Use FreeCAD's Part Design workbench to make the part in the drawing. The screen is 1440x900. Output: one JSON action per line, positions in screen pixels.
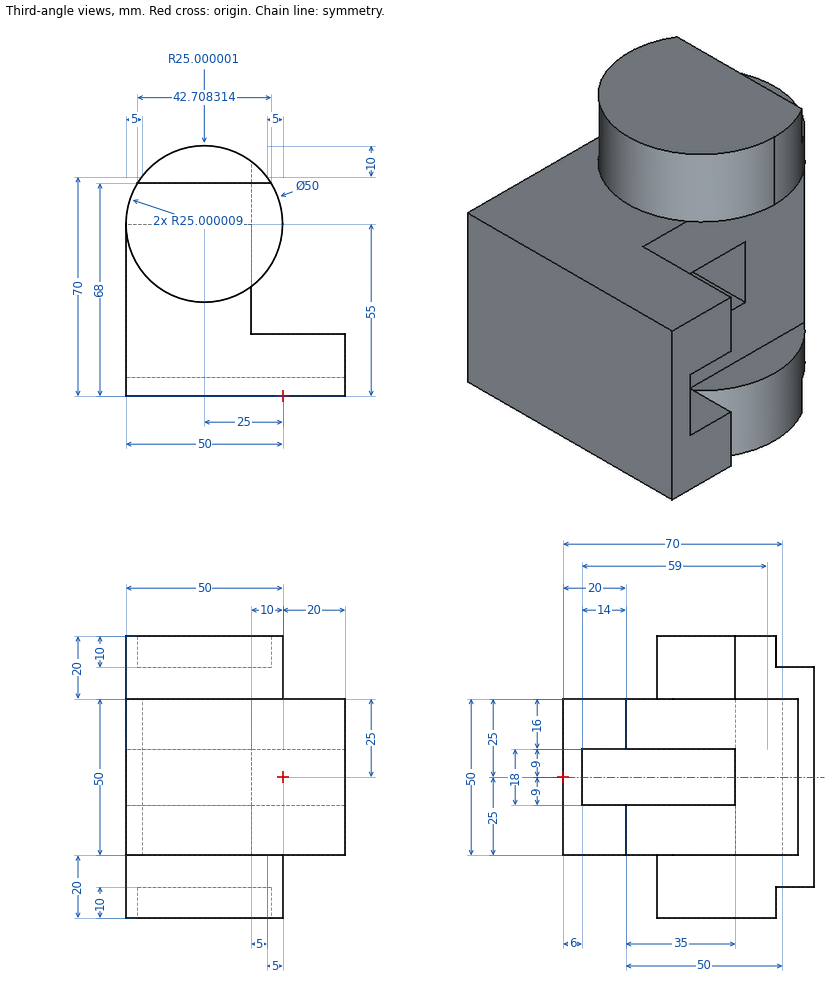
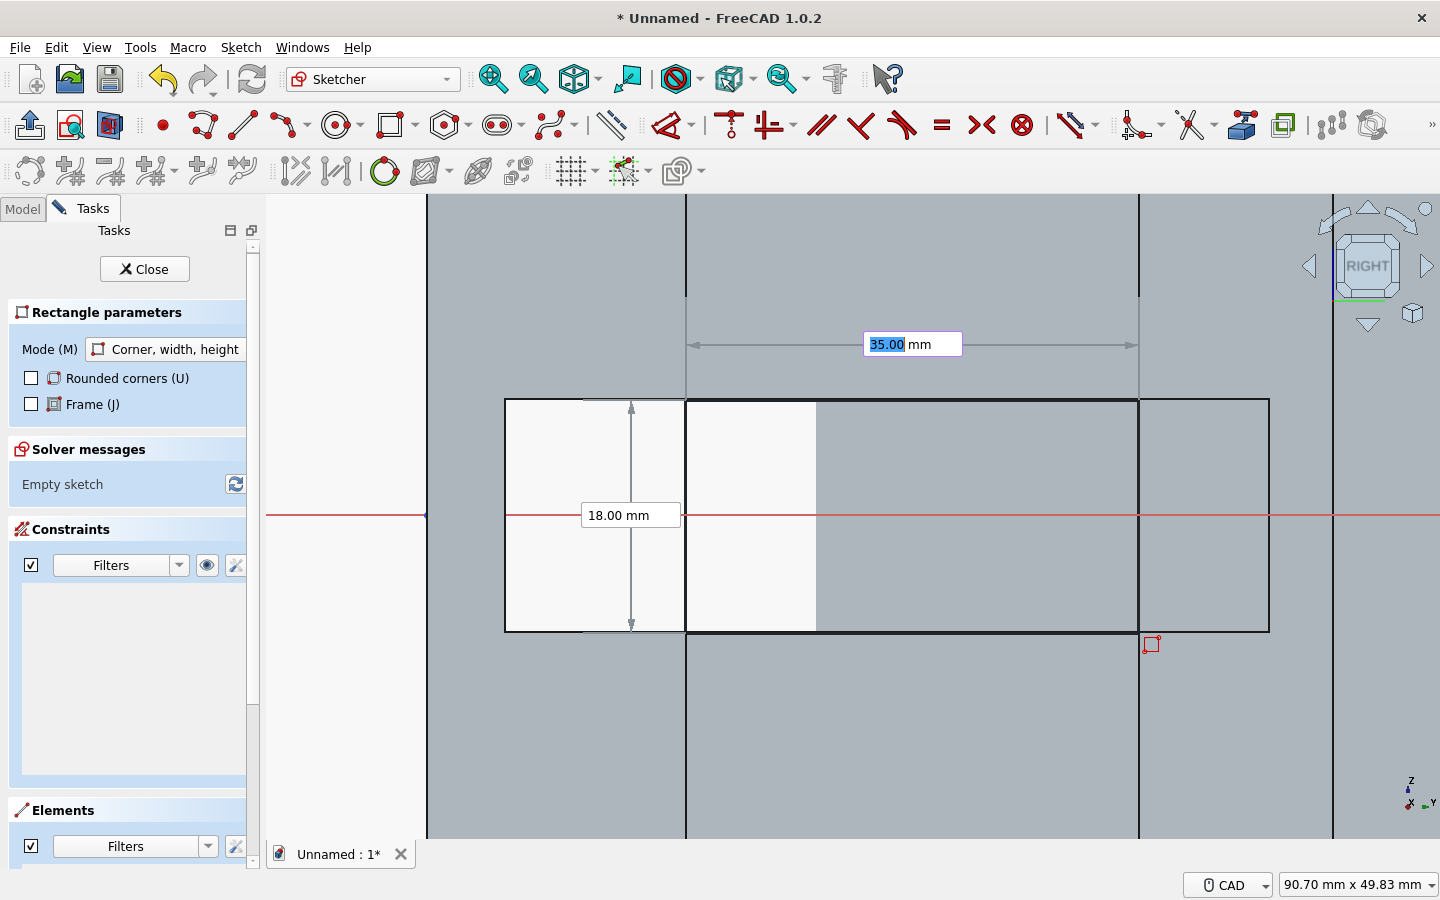
{"action": "type", "text": "35"}
{"action": "key", "text": "Tab"}
{"action": "type", "text": "18"}
{"action": "key", "text": "Return"}
{"action": "key", "text": "Escape"}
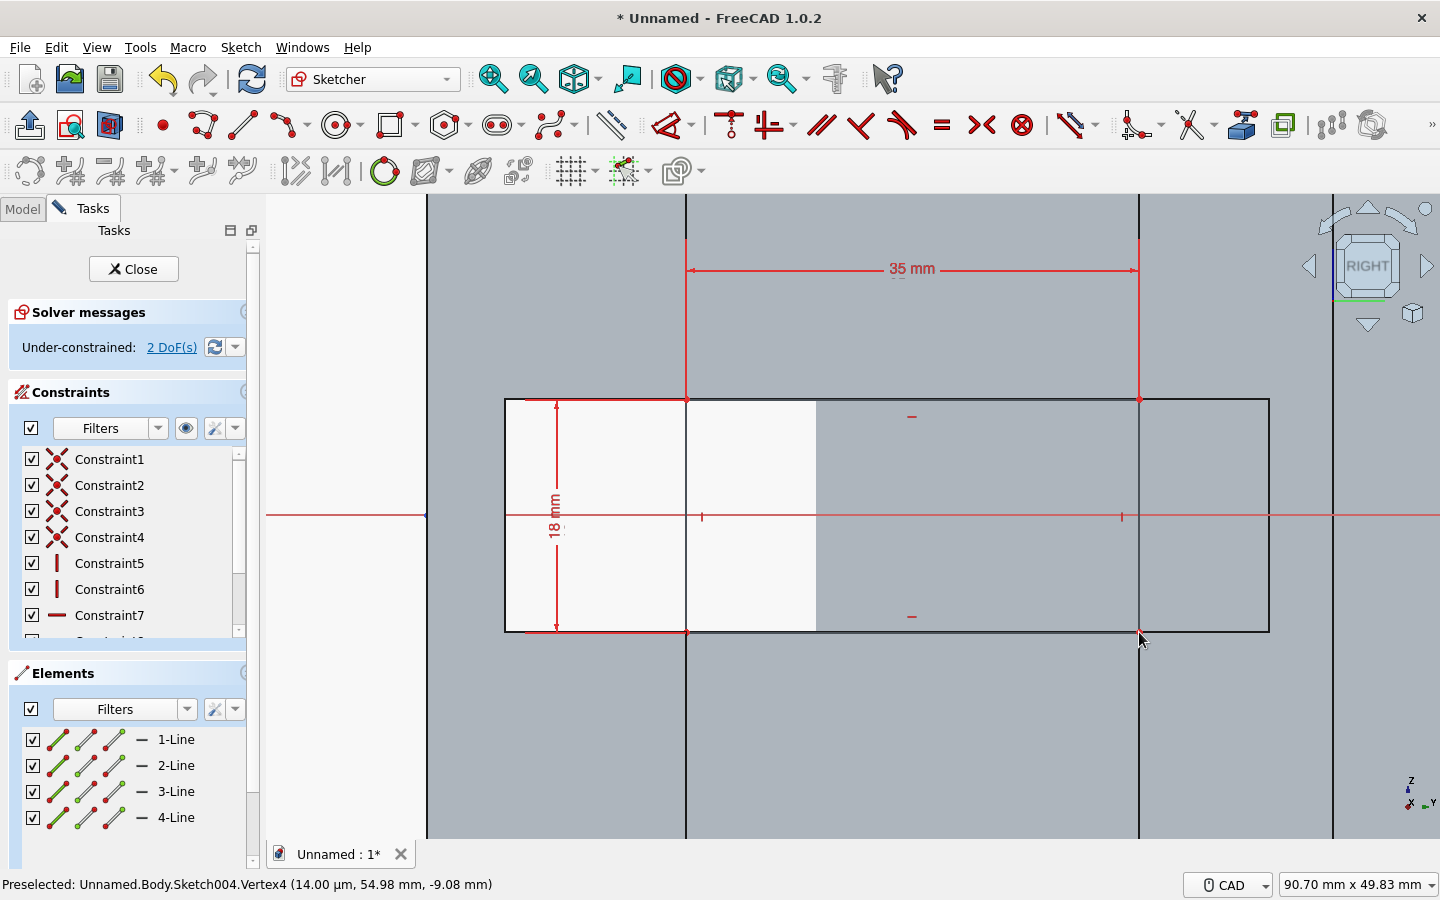
{"action": "key", "text": "d"}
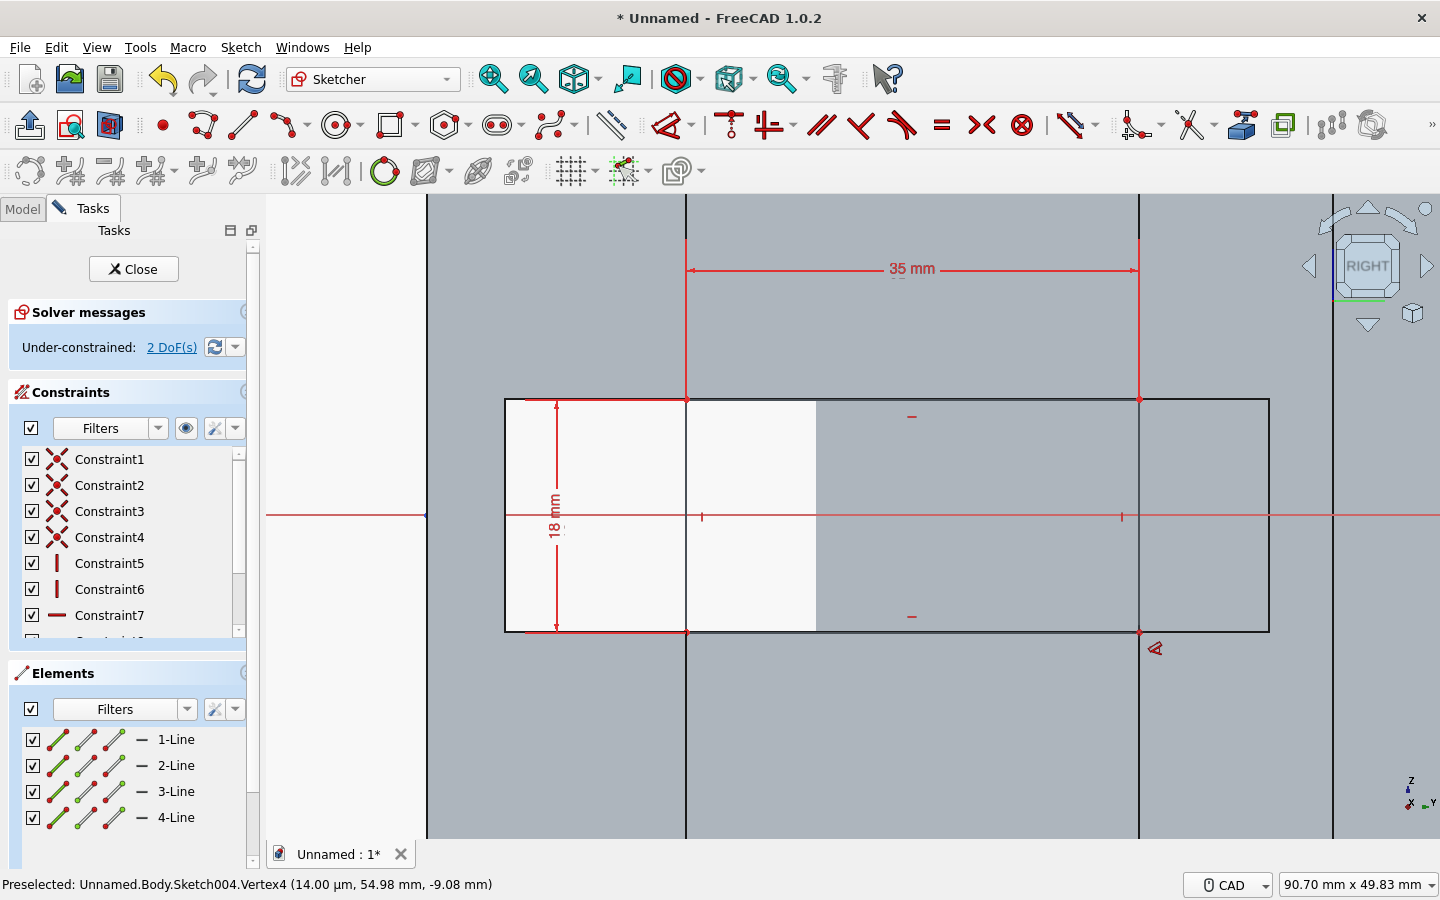
{"action": "left_click", "coordinate": [686, 400]}
{"action": "left_click", "coordinate": [393, 458]}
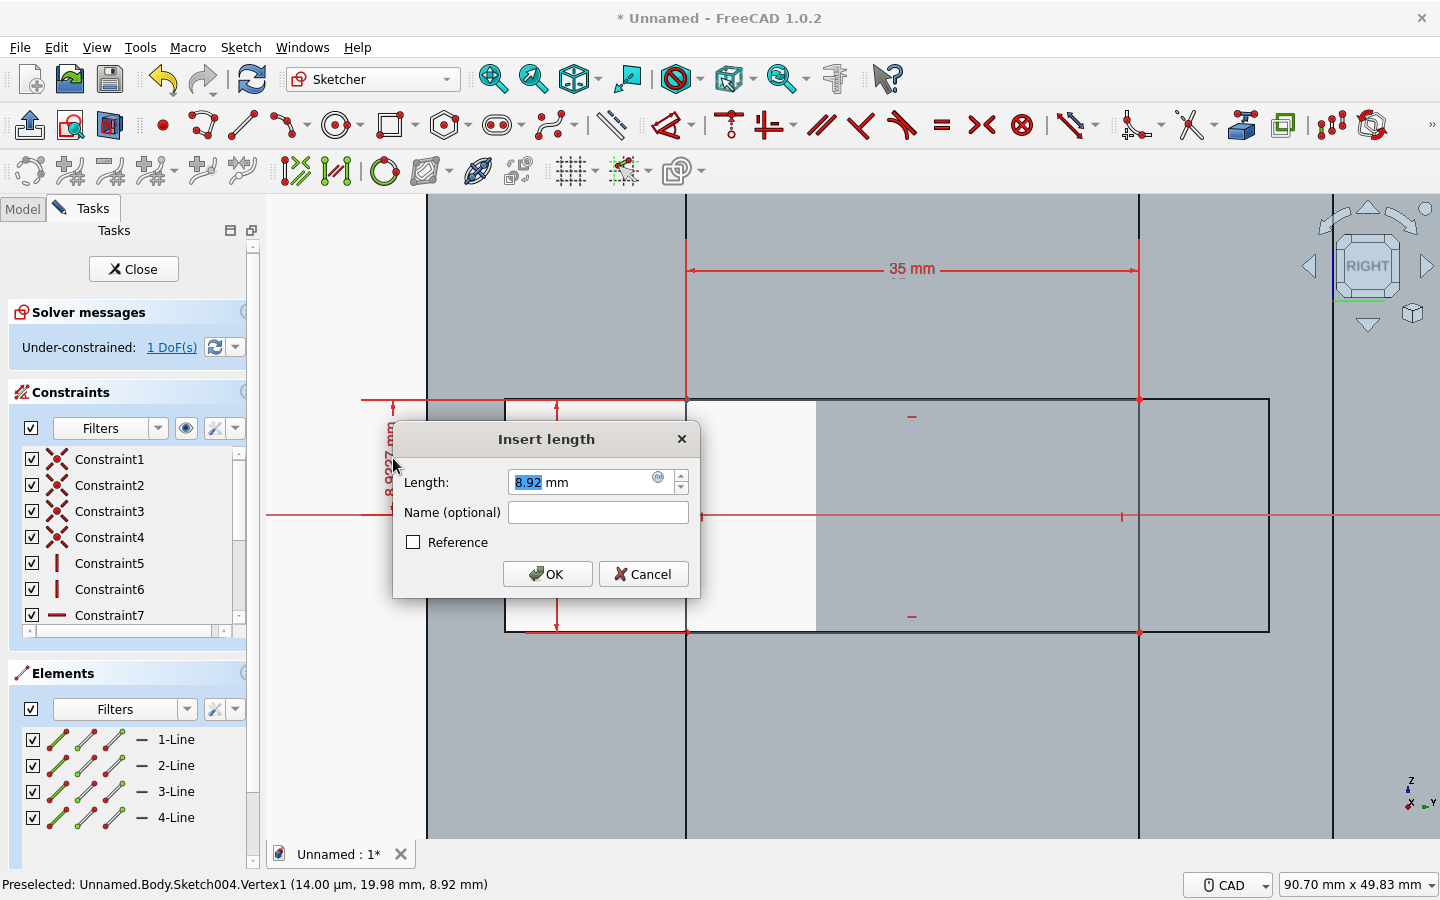
{"action": "type", "text": "9"}
{"action": "key", "text": "Return"}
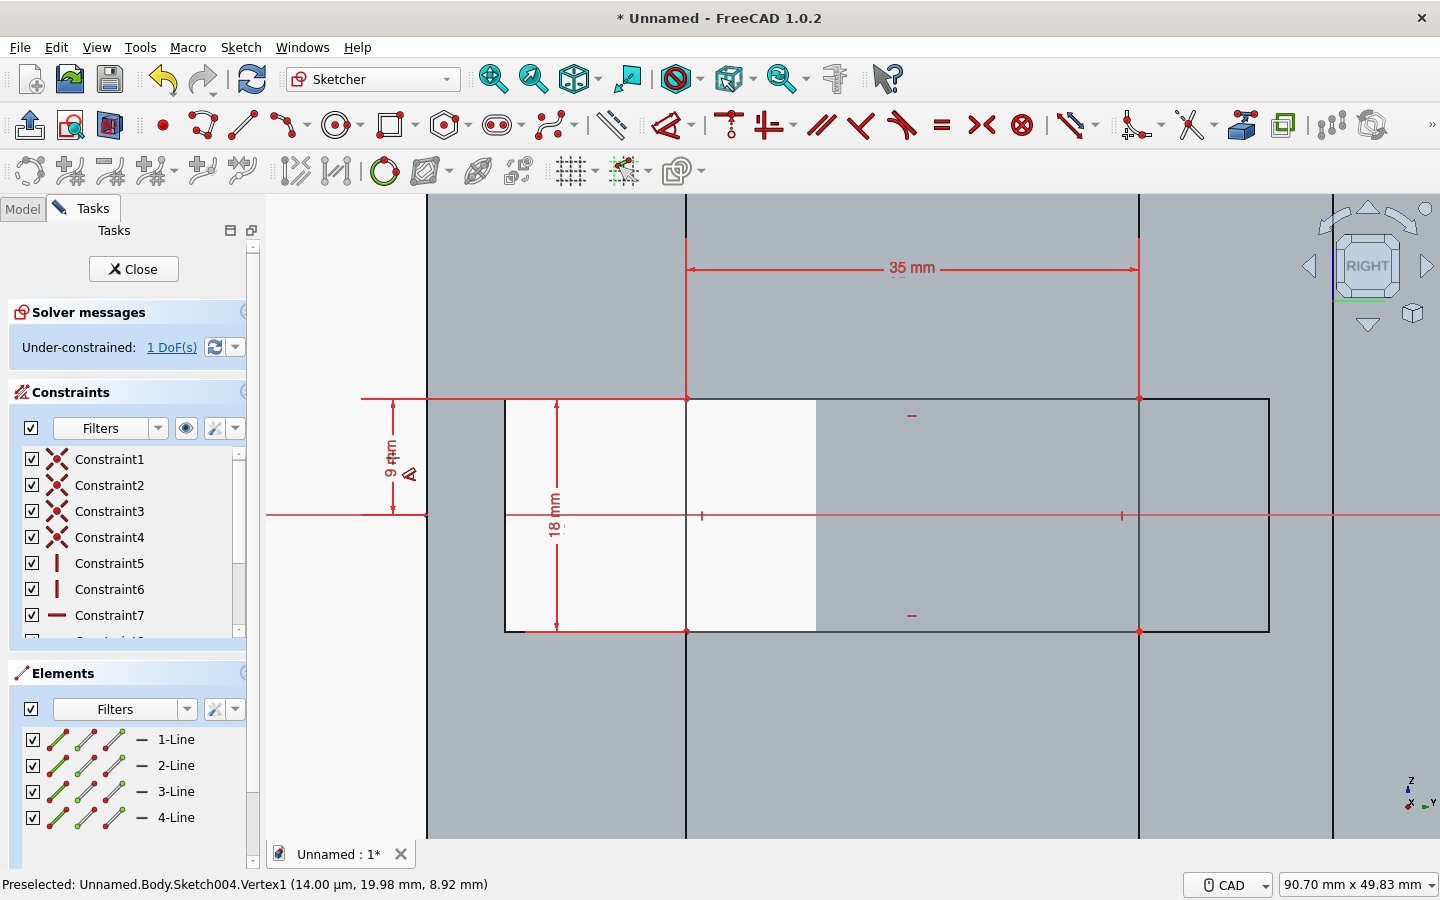
{"action": "left_click", "coordinate": [686, 399]}
{"action": "left_click", "coordinate": [557, 365]}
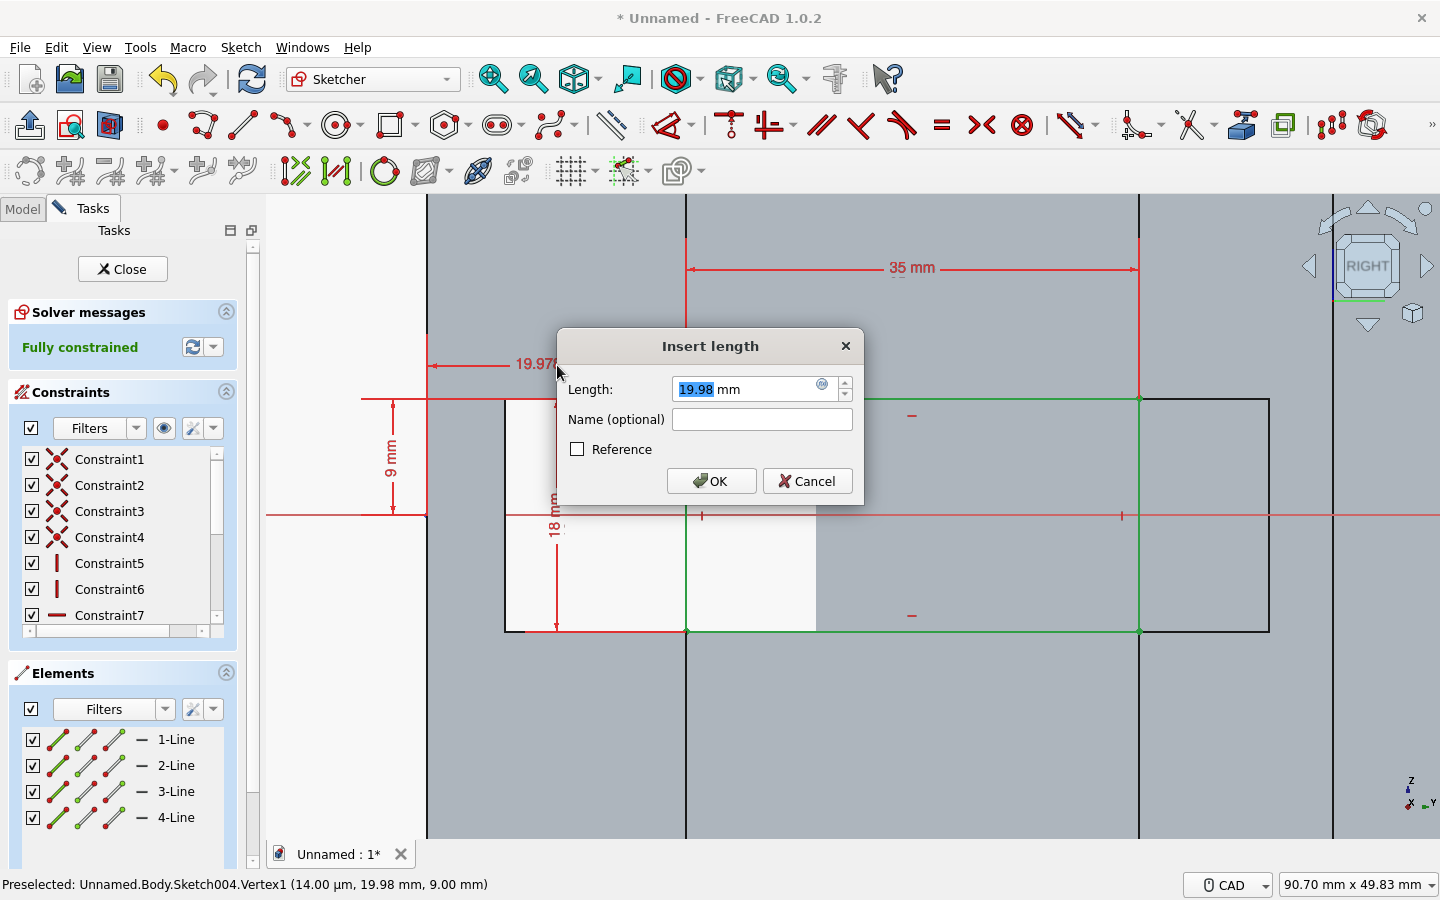
{"action": "type", "text": "20"}
{"action": "key", "text": "Return"}
{"action": "key", "text": "Escape"}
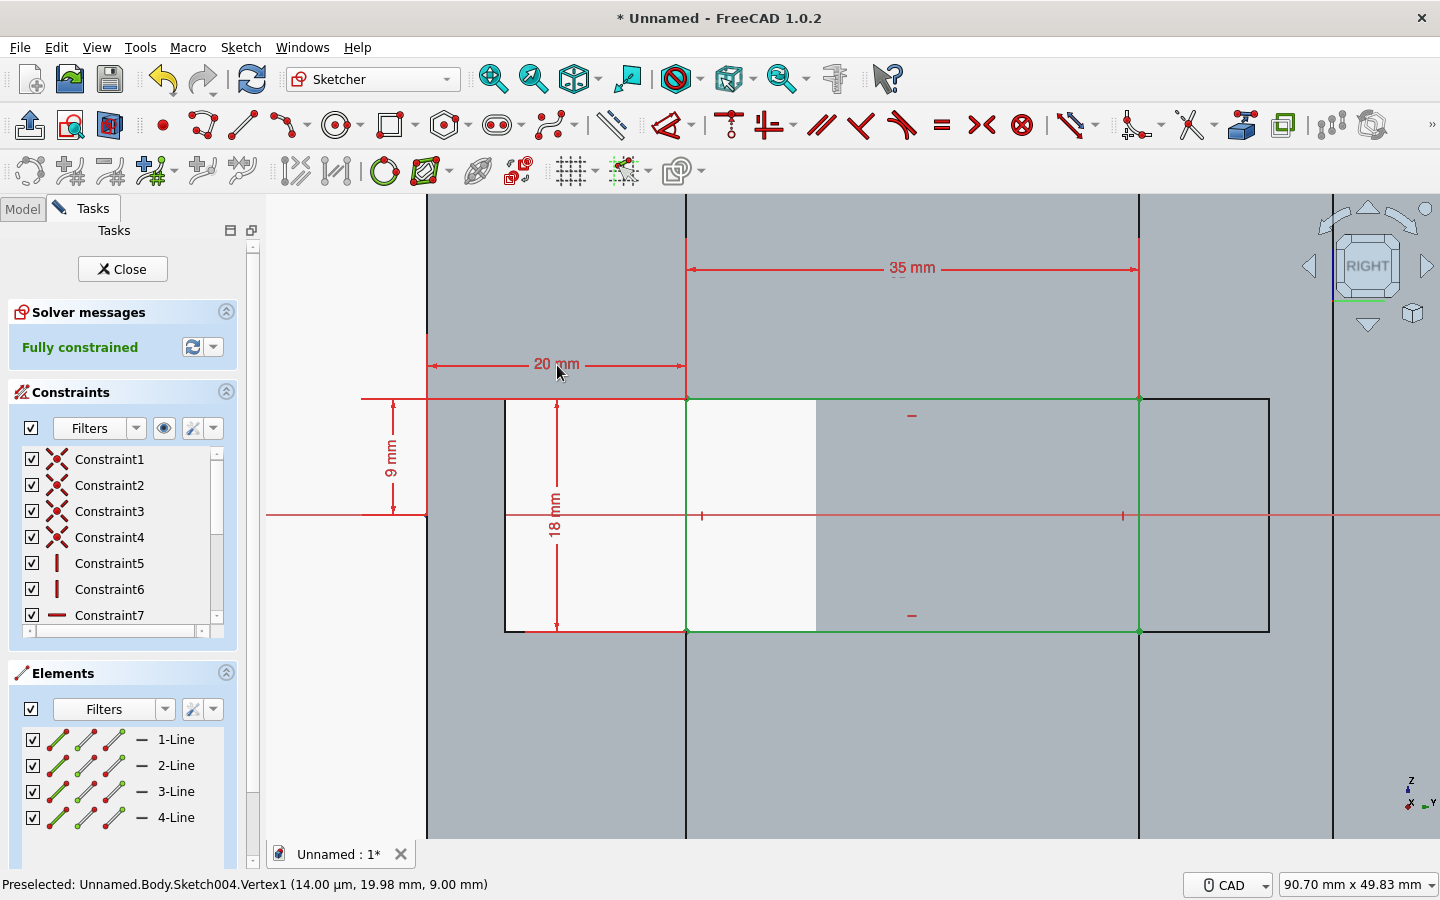
{"action": "left_click", "coordinate": [123, 269]}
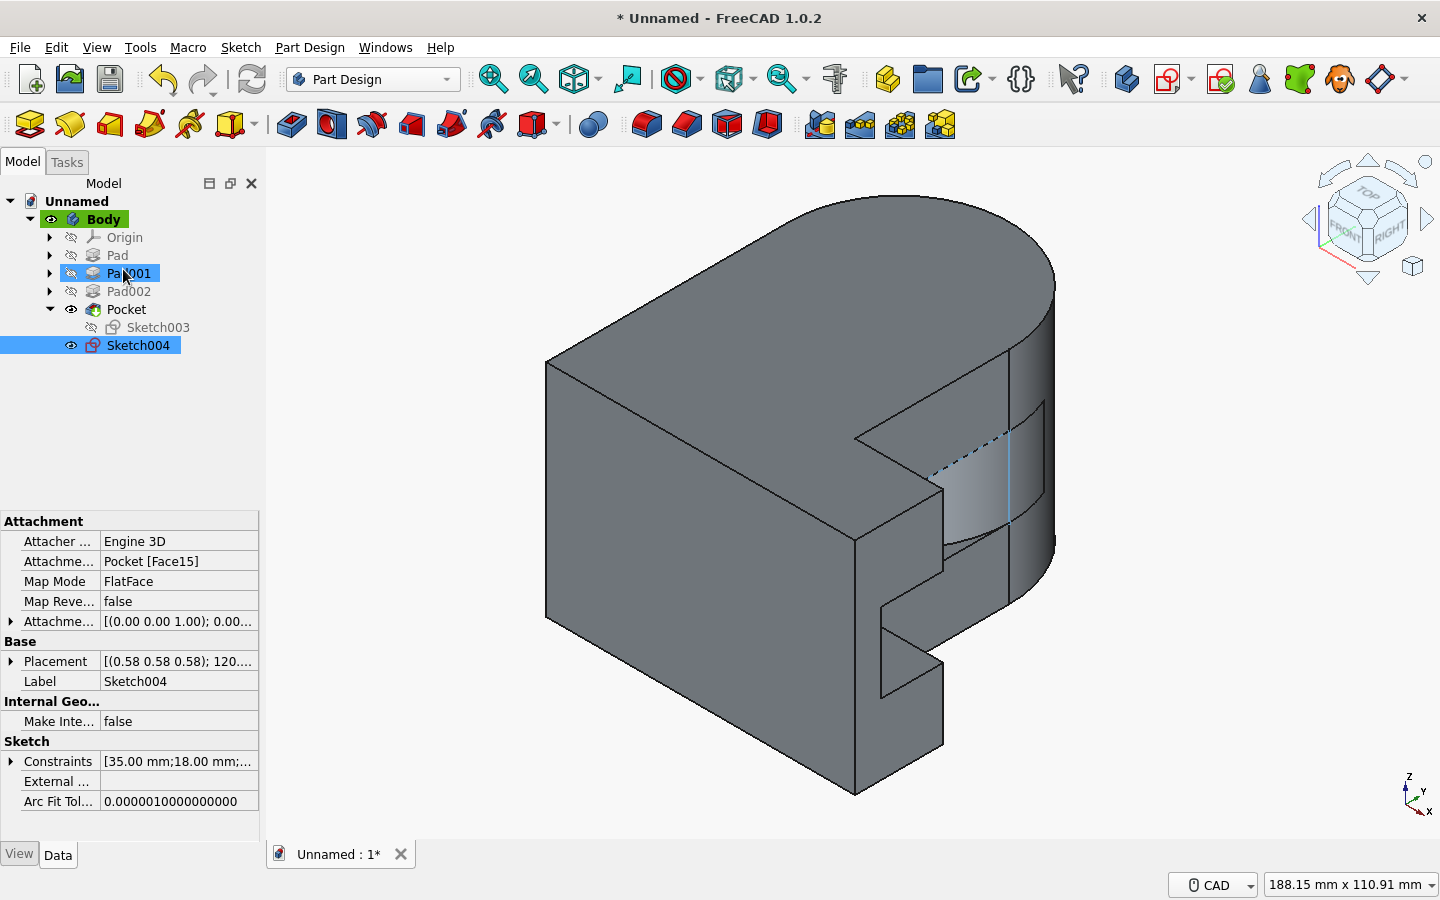
{"action": "left_click", "coordinate": [292, 124]}